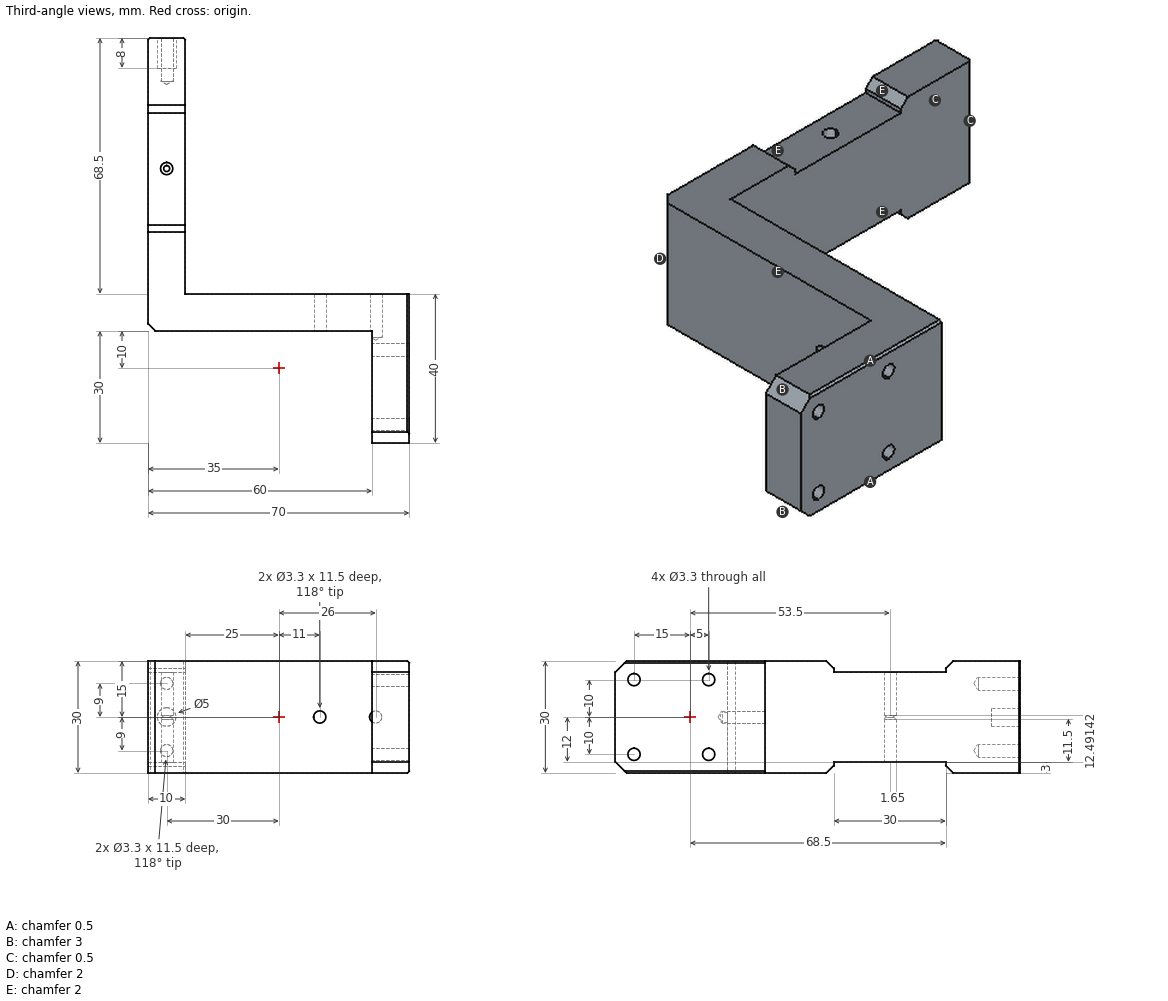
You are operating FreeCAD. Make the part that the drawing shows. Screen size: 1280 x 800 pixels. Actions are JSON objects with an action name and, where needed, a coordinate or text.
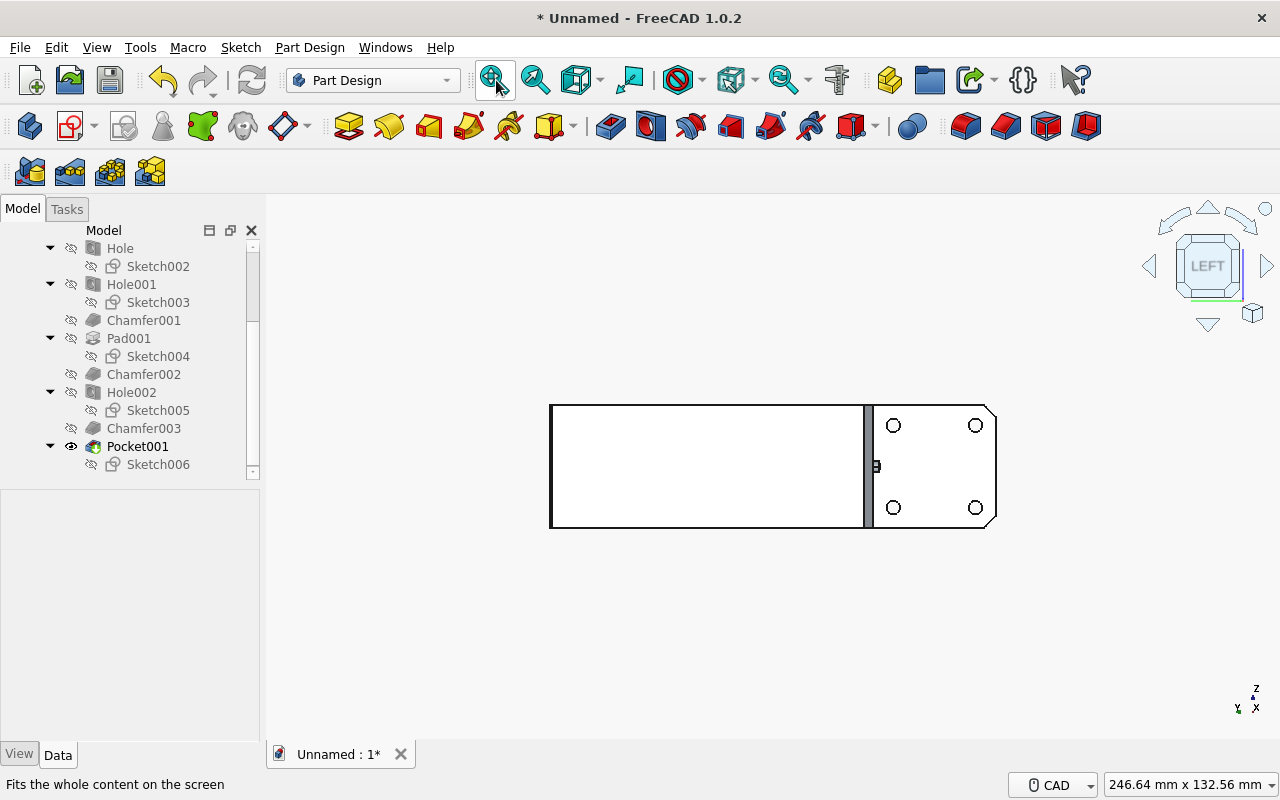
{"action": "left_click", "coordinate": [798, 465]}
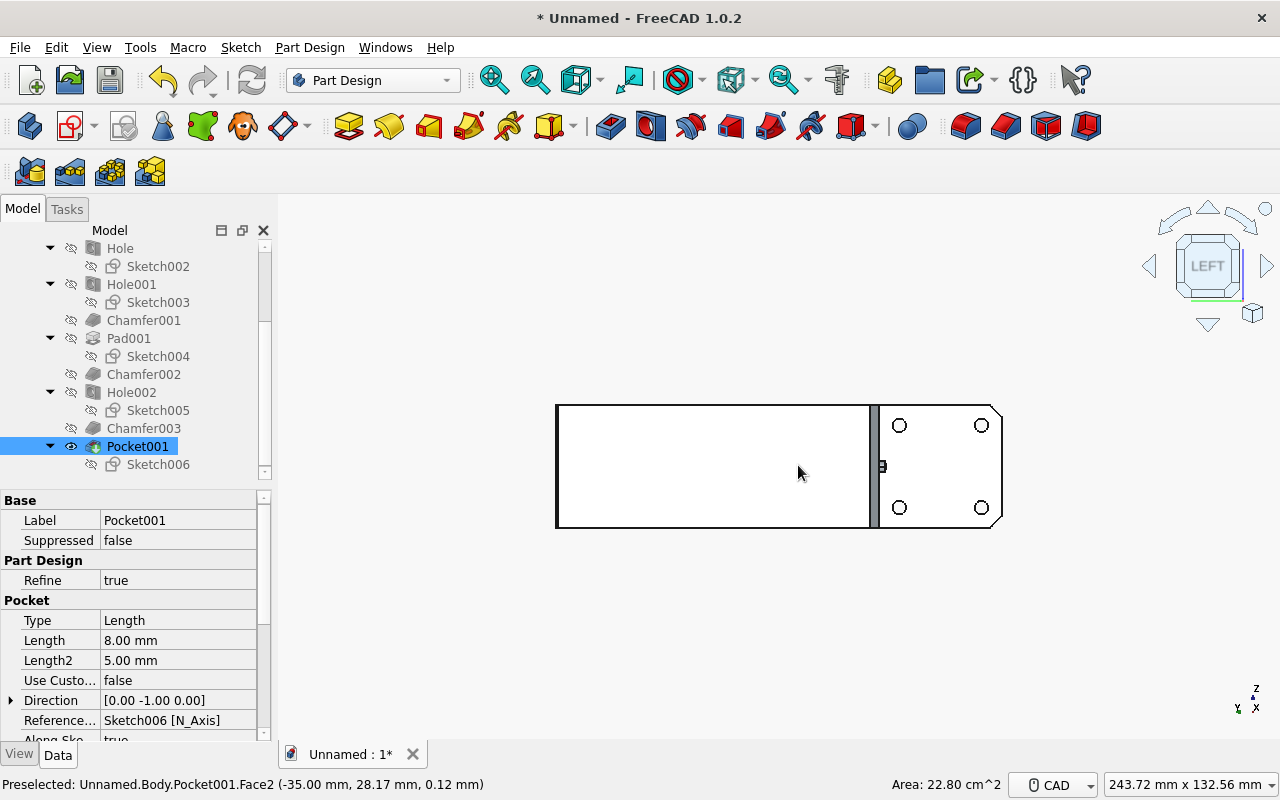
{"action": "left_click", "coordinate": [70, 126]}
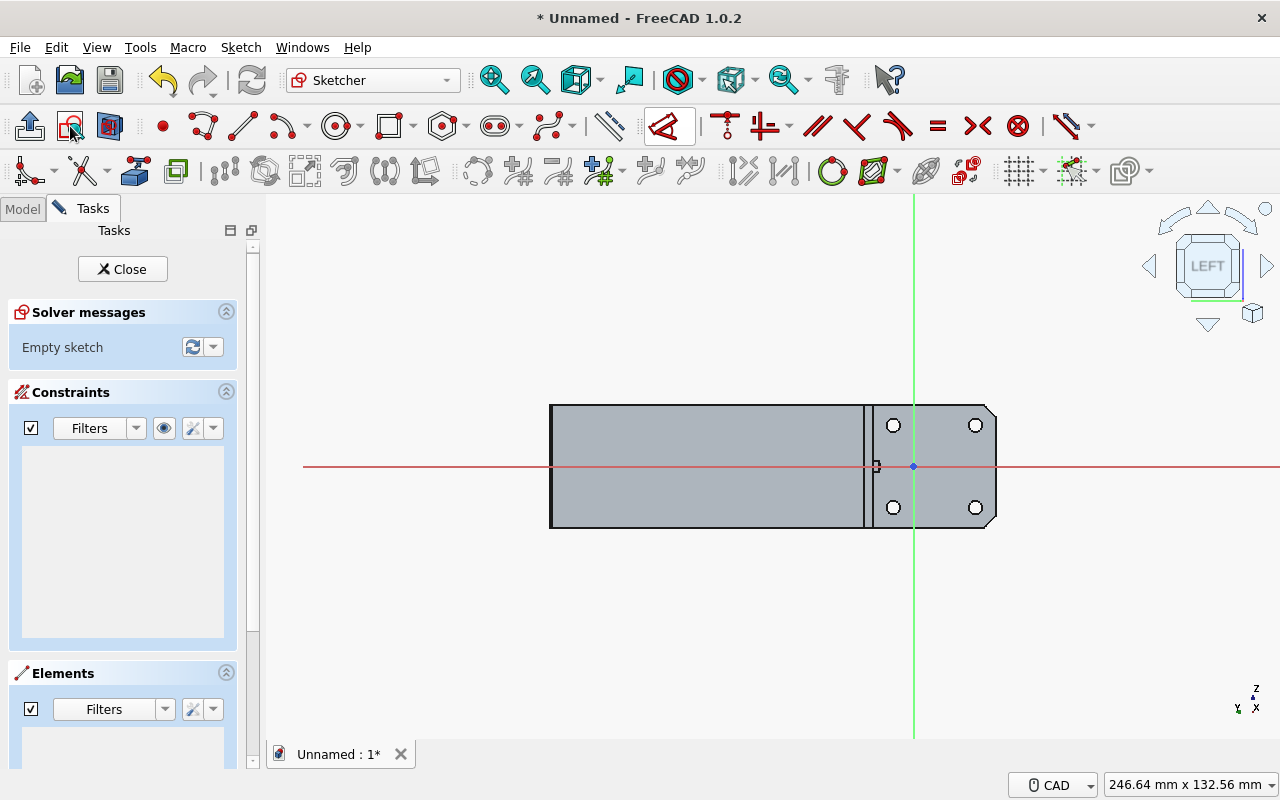
{"action": "scroll", "coordinate": [829, 522], "scroll_direction": "up", "scroll_amount": 4}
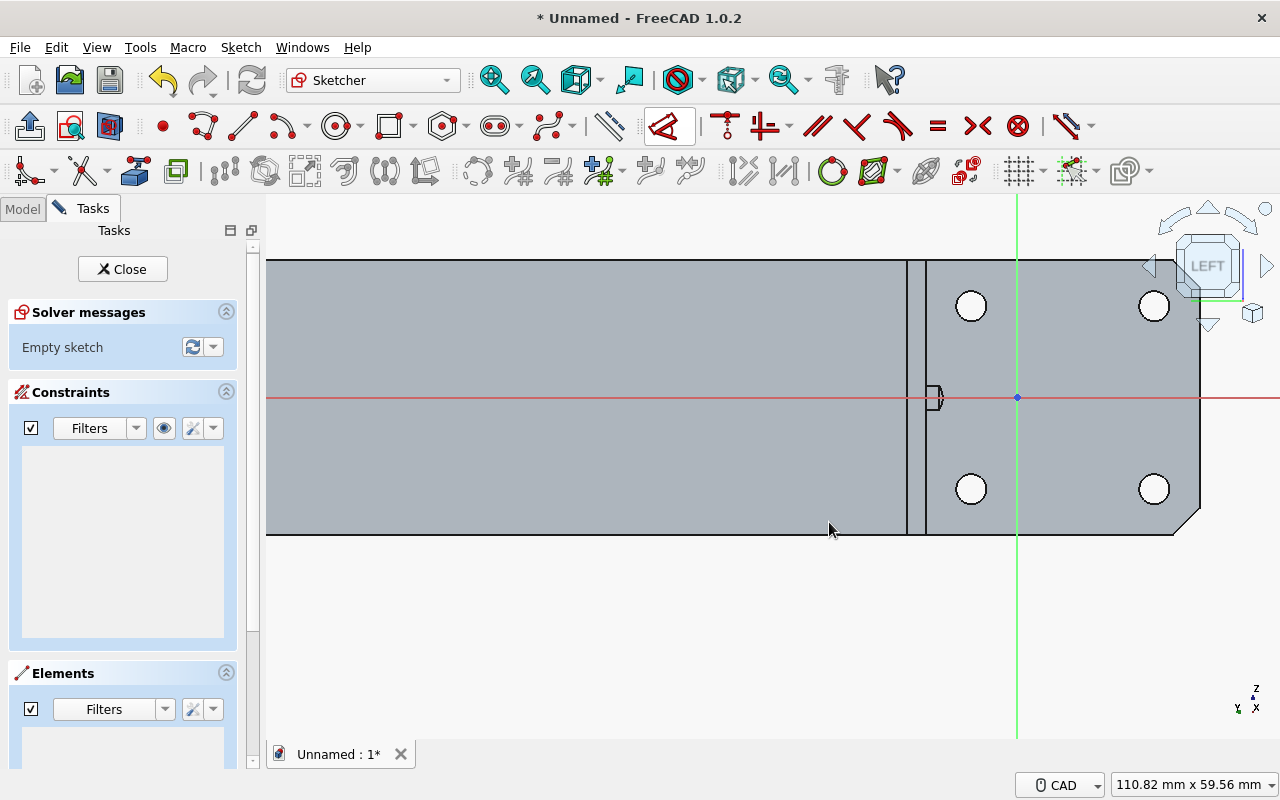
{"action": "left_click", "coordinate": [390, 126]}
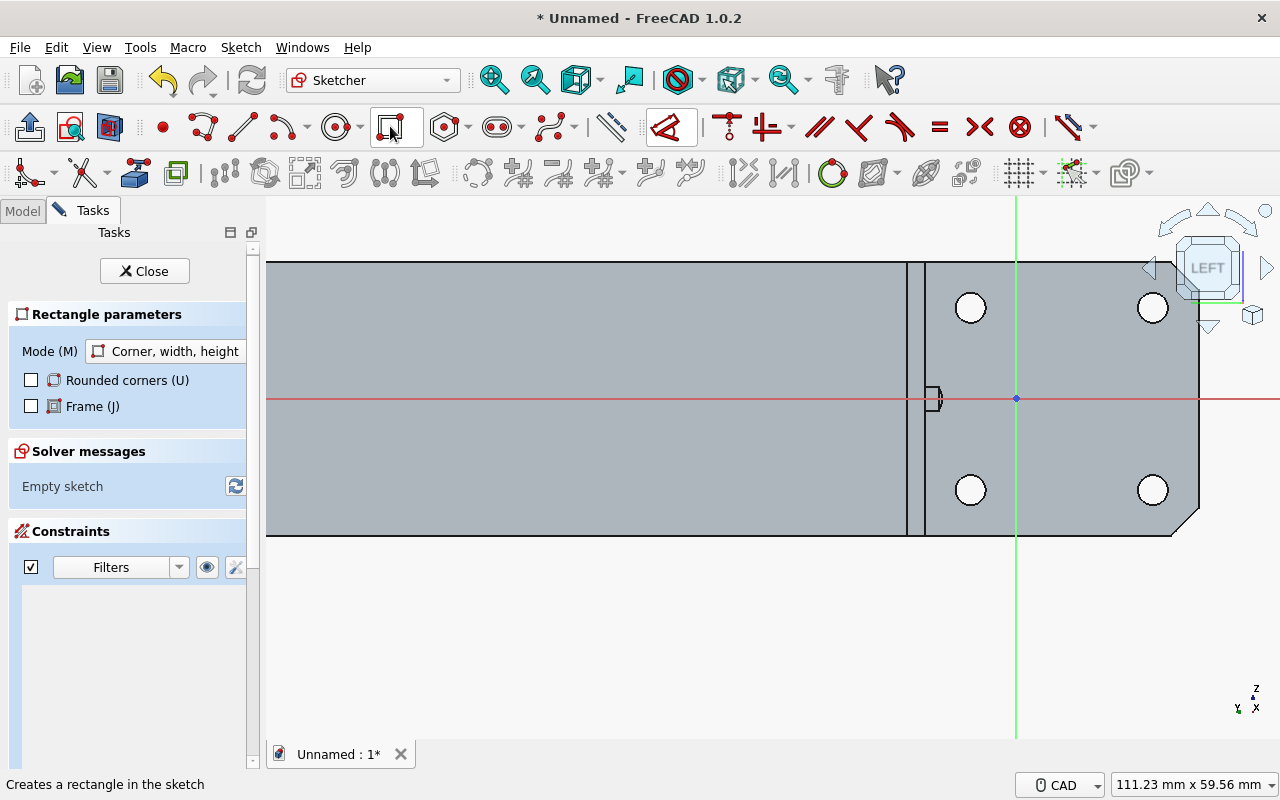
{"action": "left_click", "coordinate": [392, 508]}
{"action": "left_click", "coordinate": [665, 536]}
{"action": "key", "text": "Escape"}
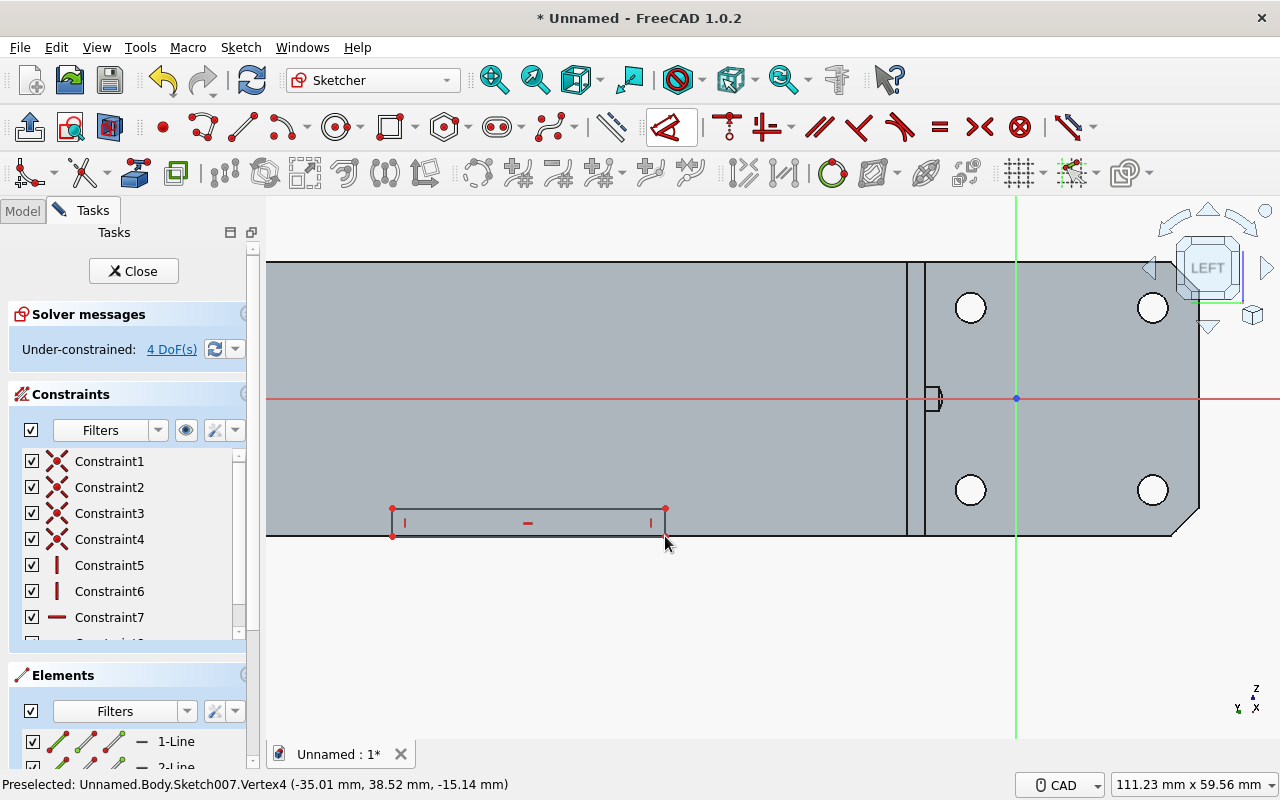
{"action": "scroll", "coordinate": [392, 520], "scroll_direction": "up", "scroll_amount": 2}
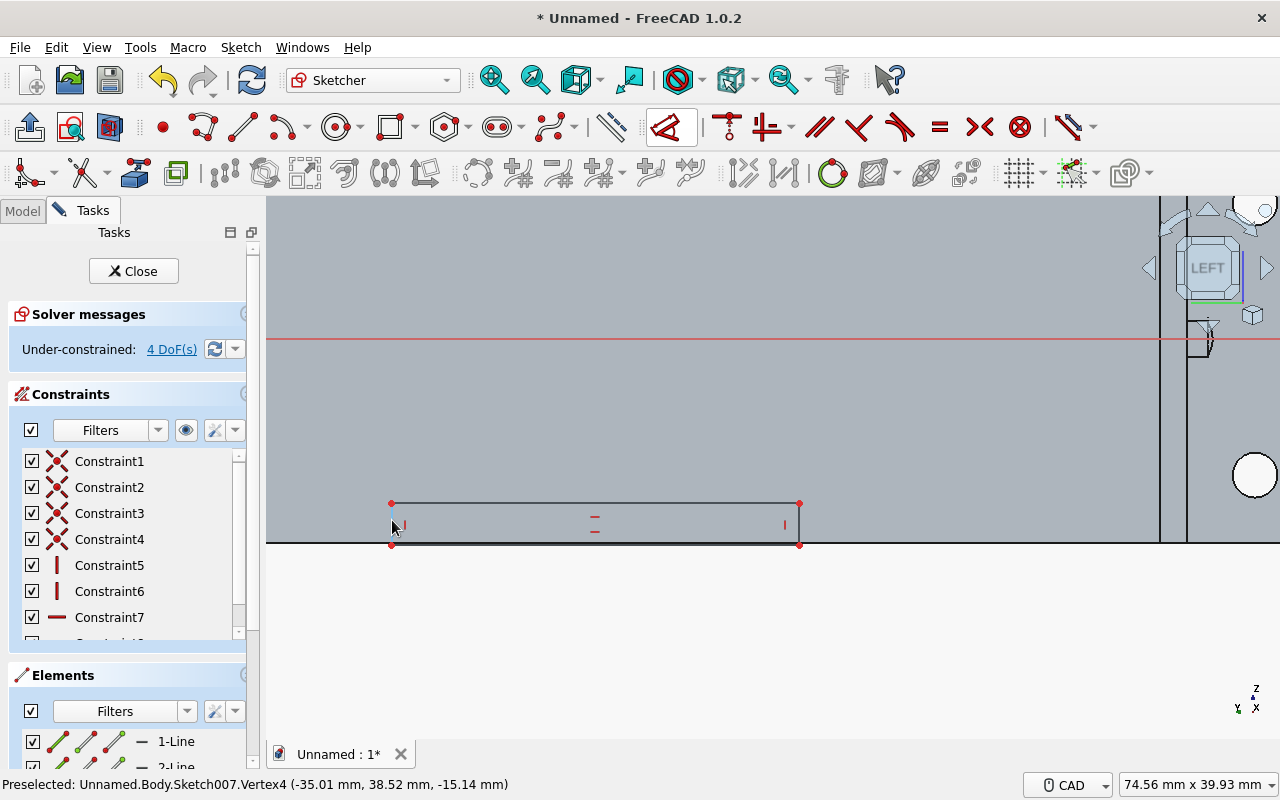
{"action": "left_click", "coordinate": [392, 520]}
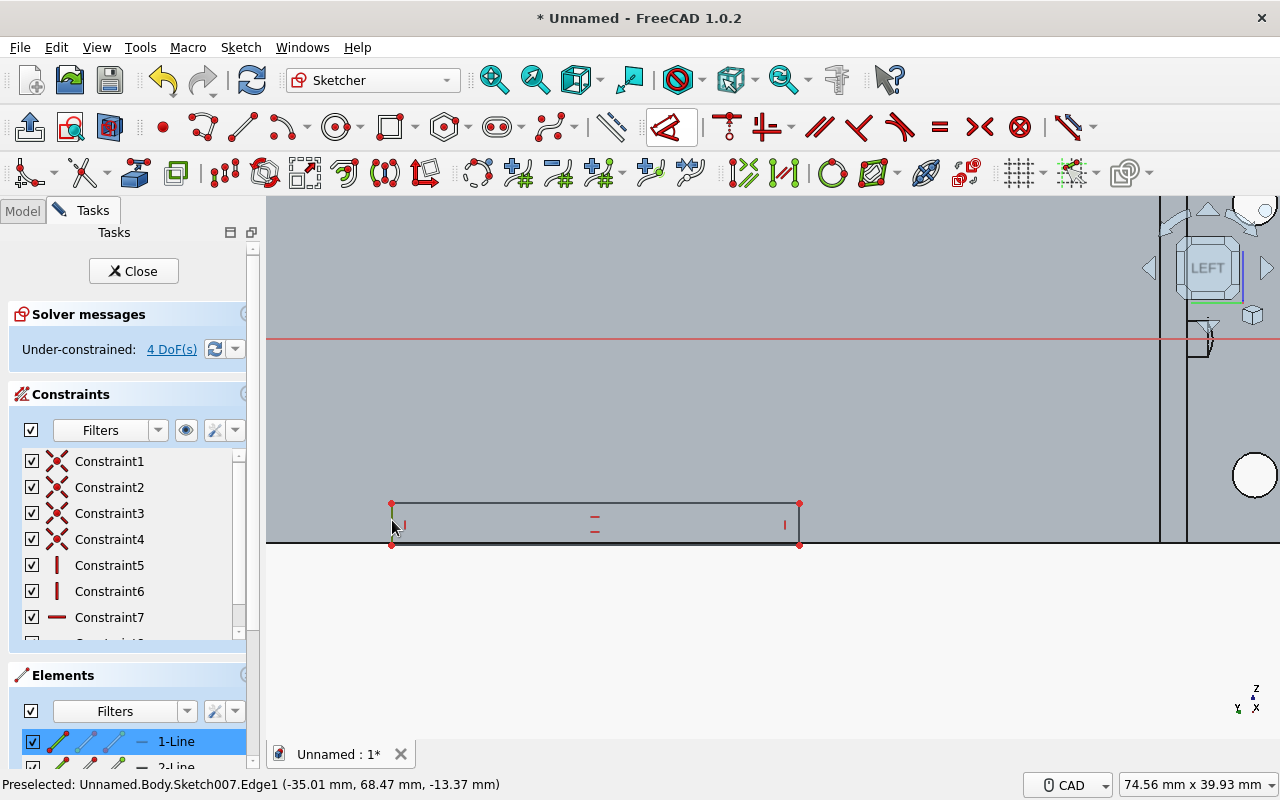
{"action": "key", "text": "i"}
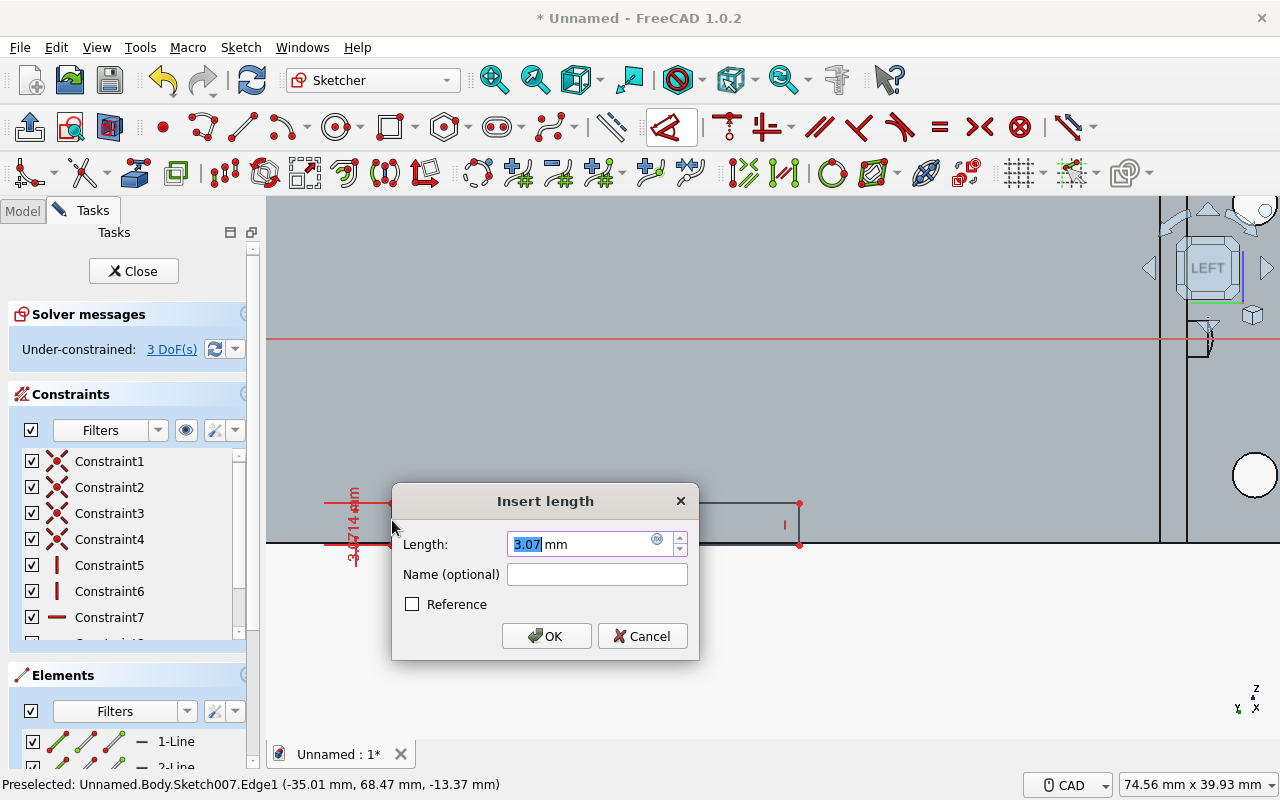
{"action": "type", "text": "3"}
{"action": "key", "text": "Return"}